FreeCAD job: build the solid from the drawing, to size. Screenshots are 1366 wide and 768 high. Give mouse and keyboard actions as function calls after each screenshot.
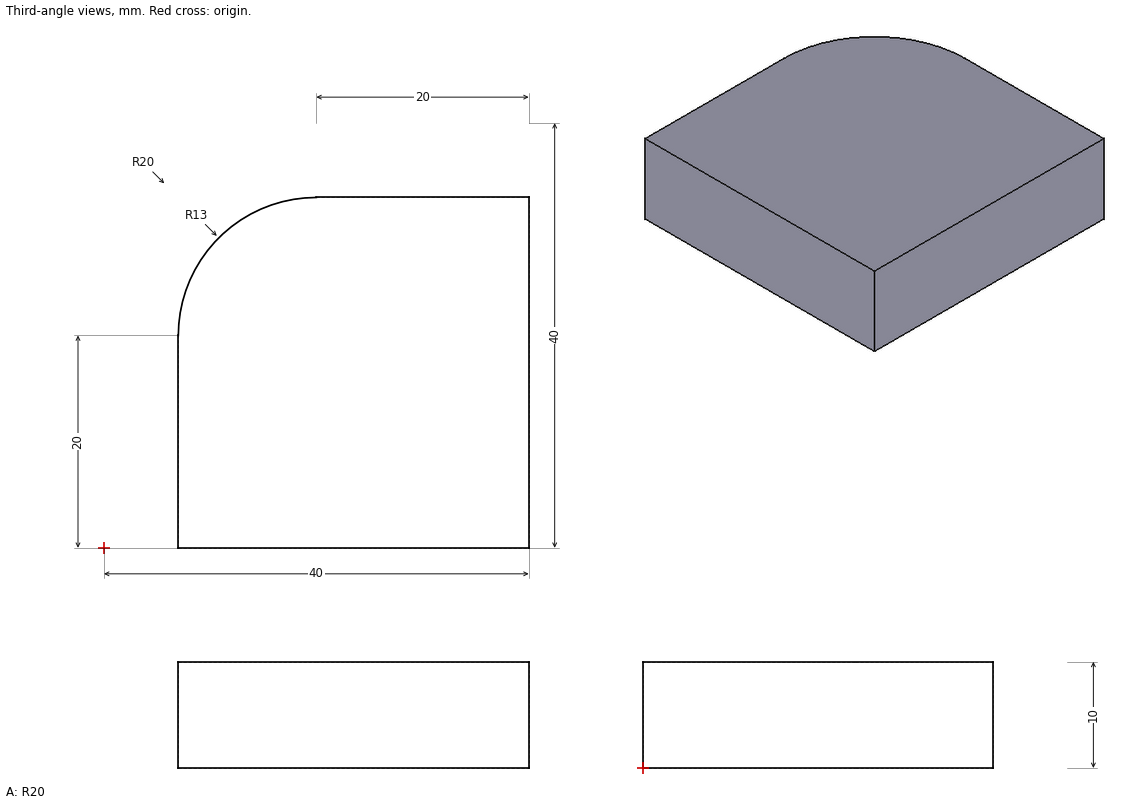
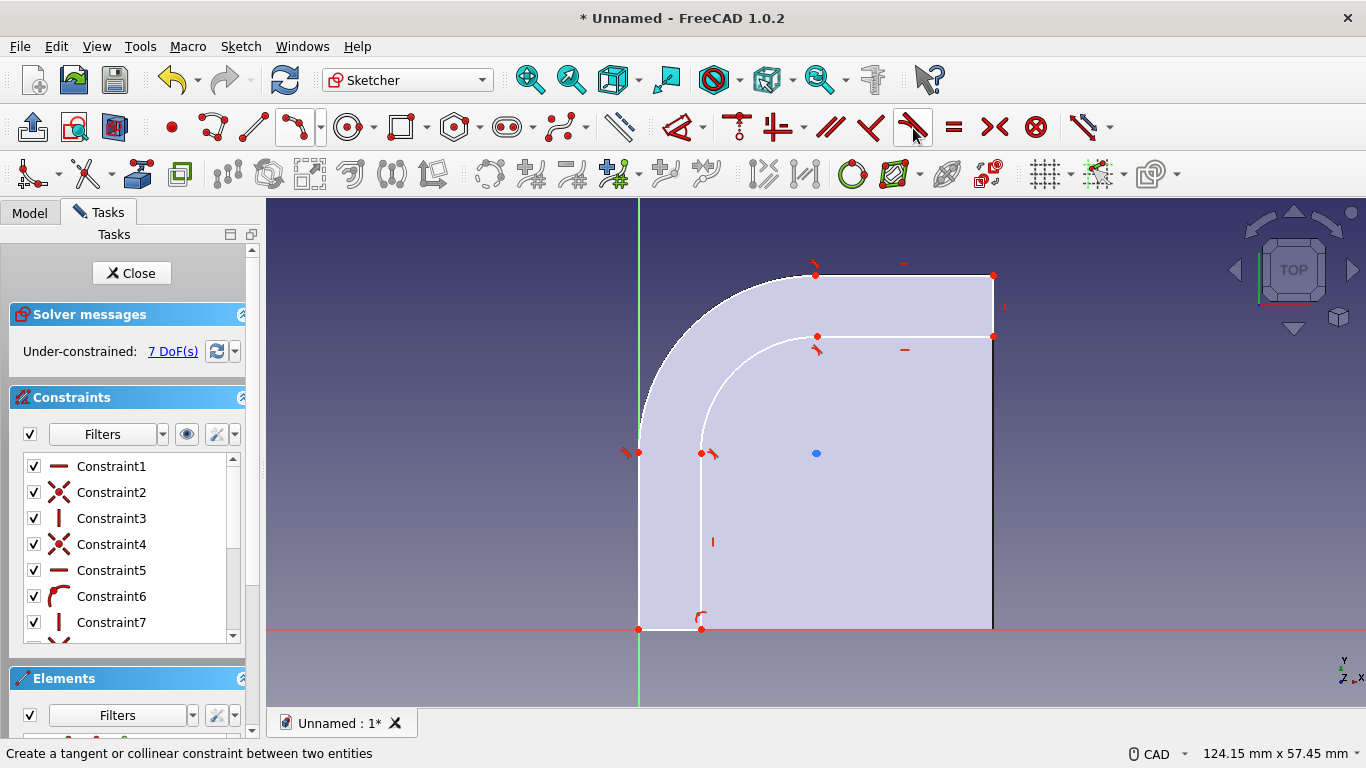
click(639, 577)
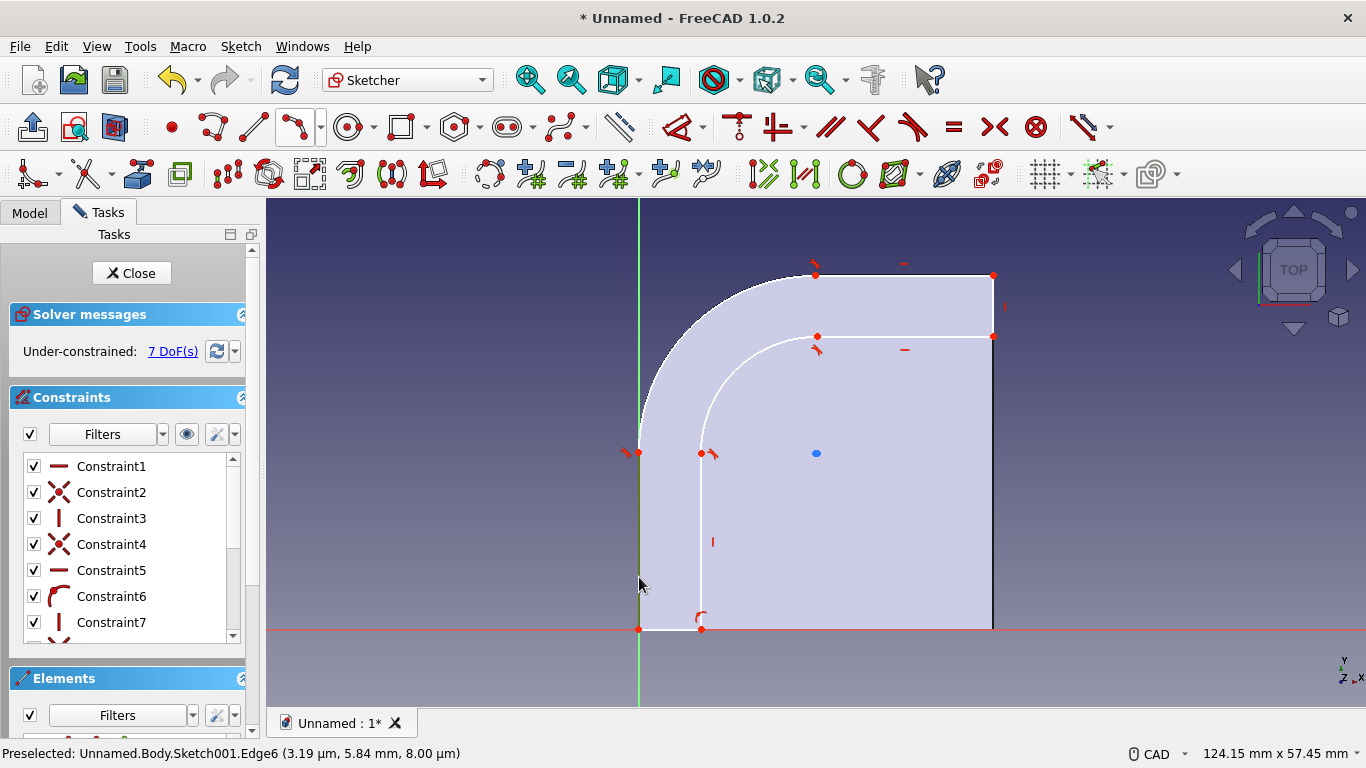
key(v)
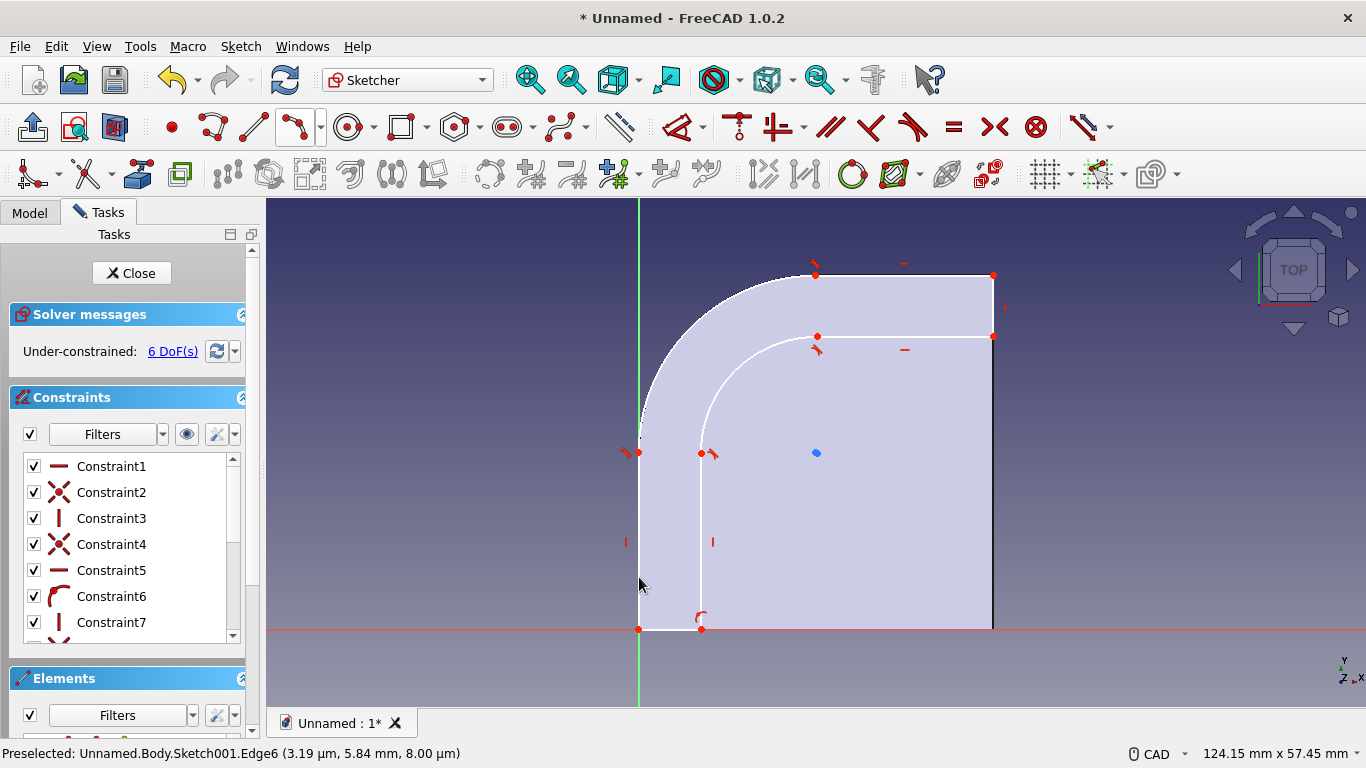
click(764, 350)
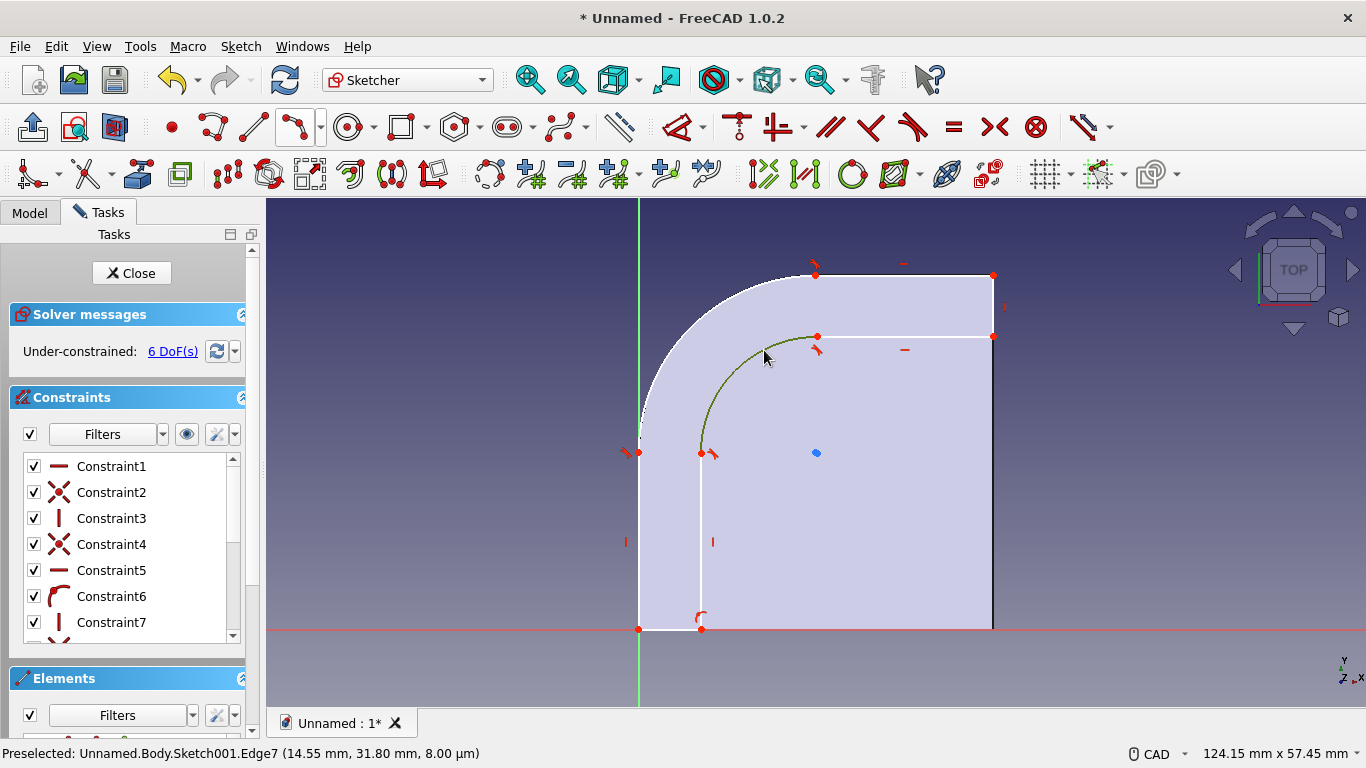
click(736, 295)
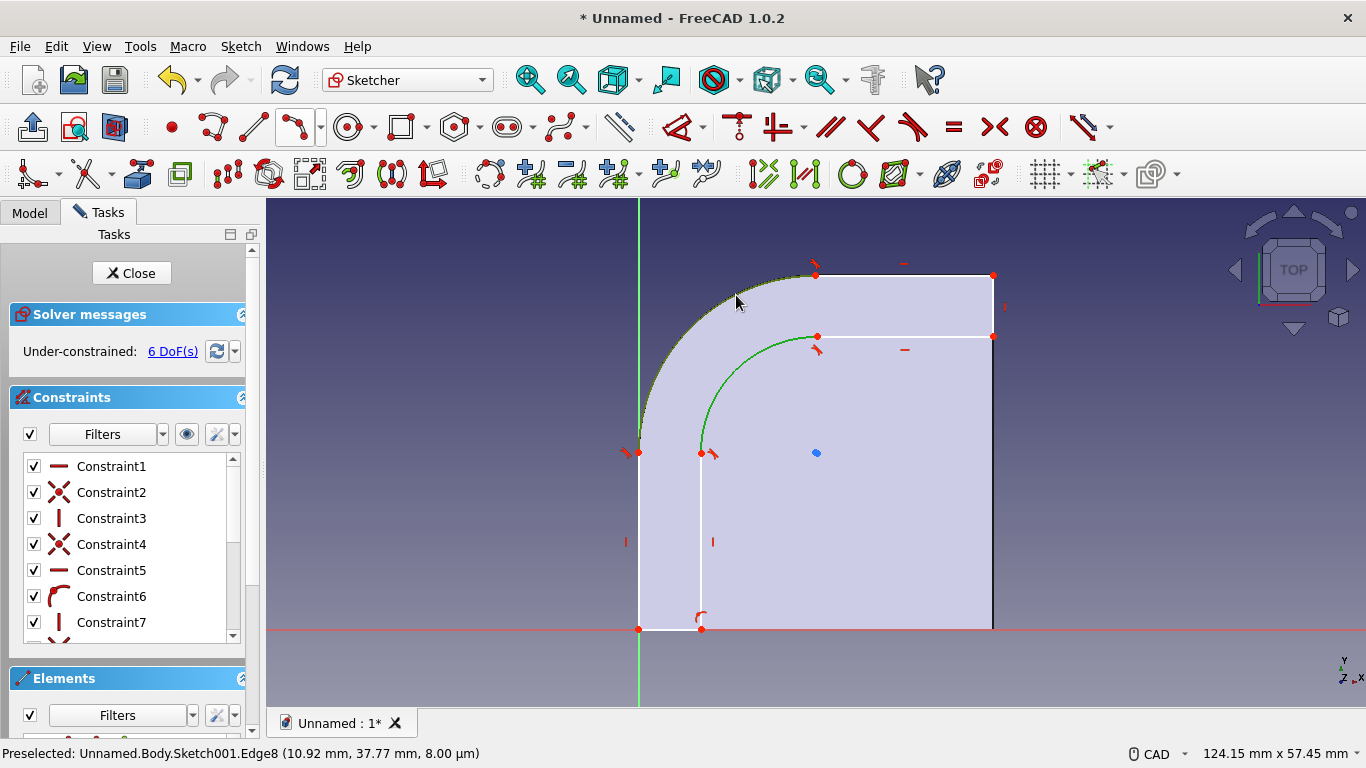
click(737, 128)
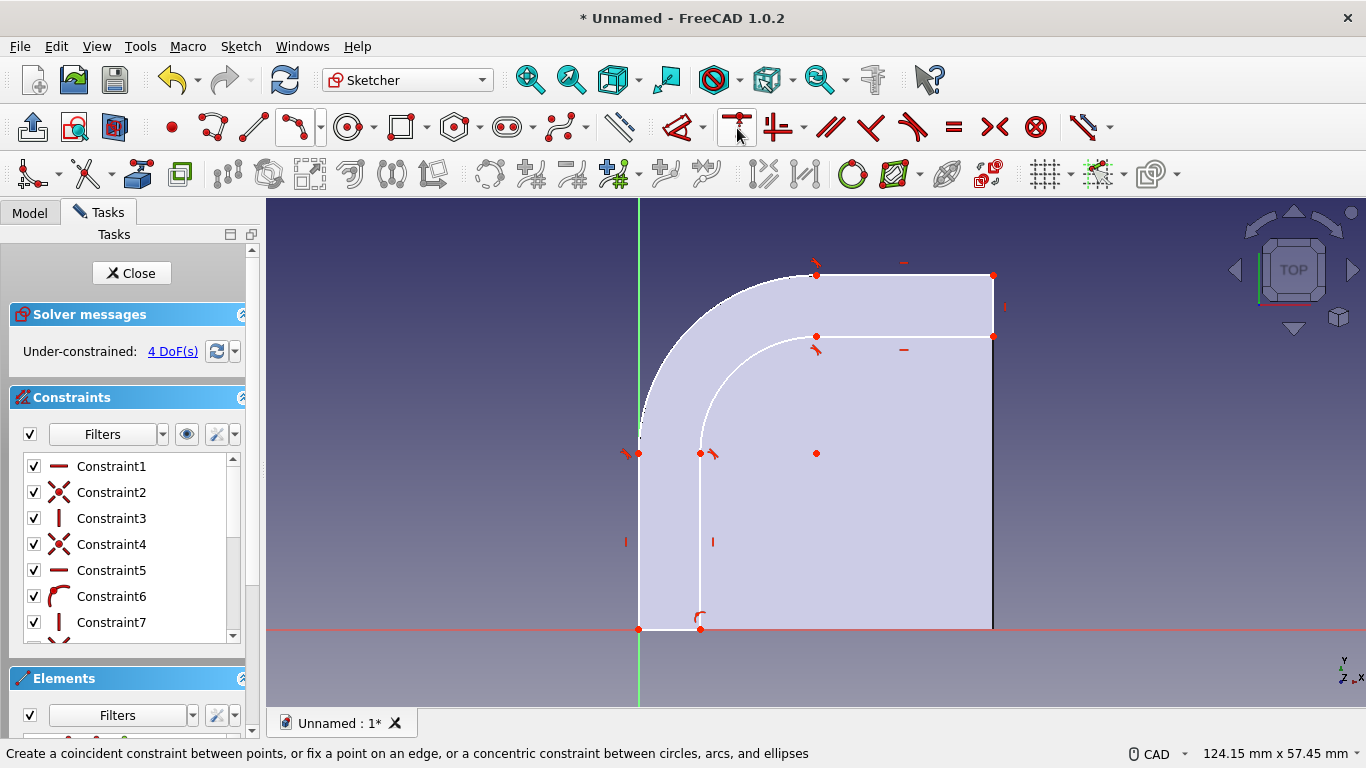
click(676, 128)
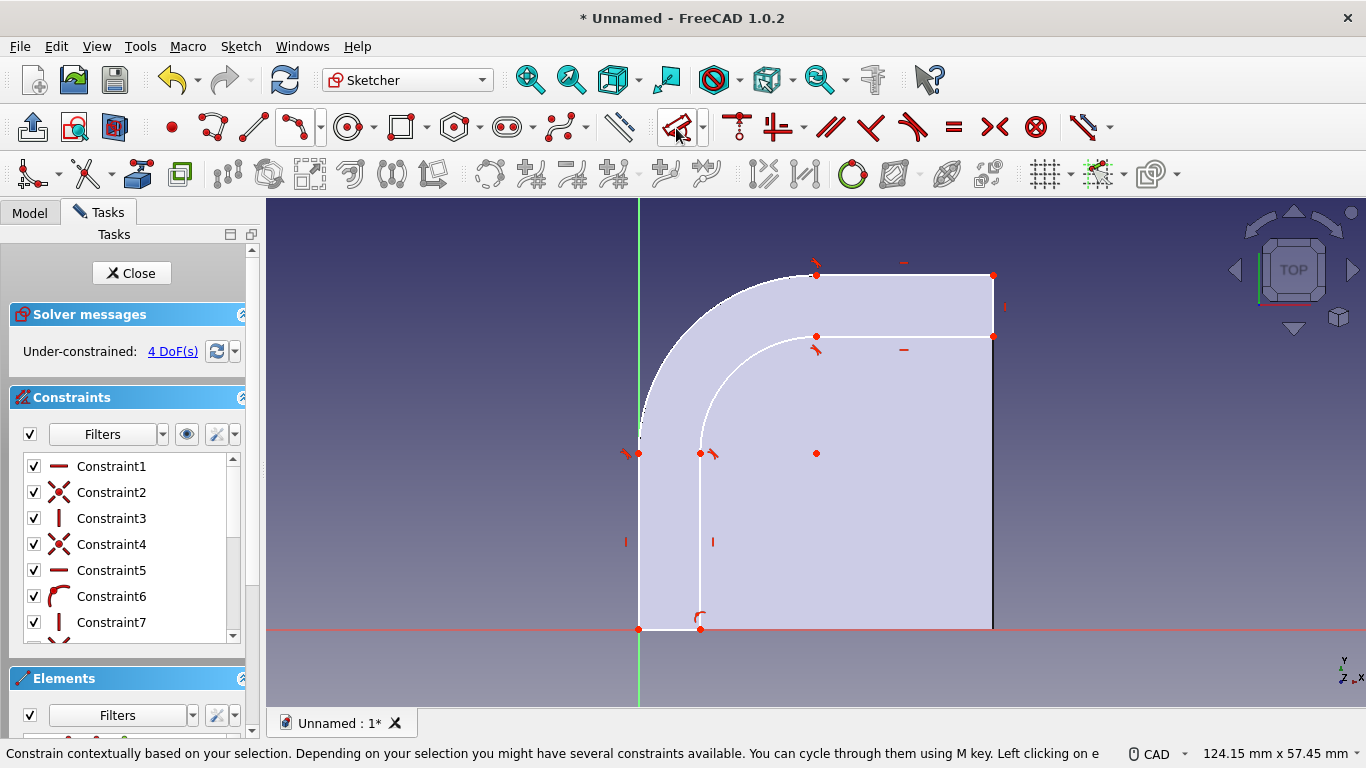
click(764, 350)
click(749, 321)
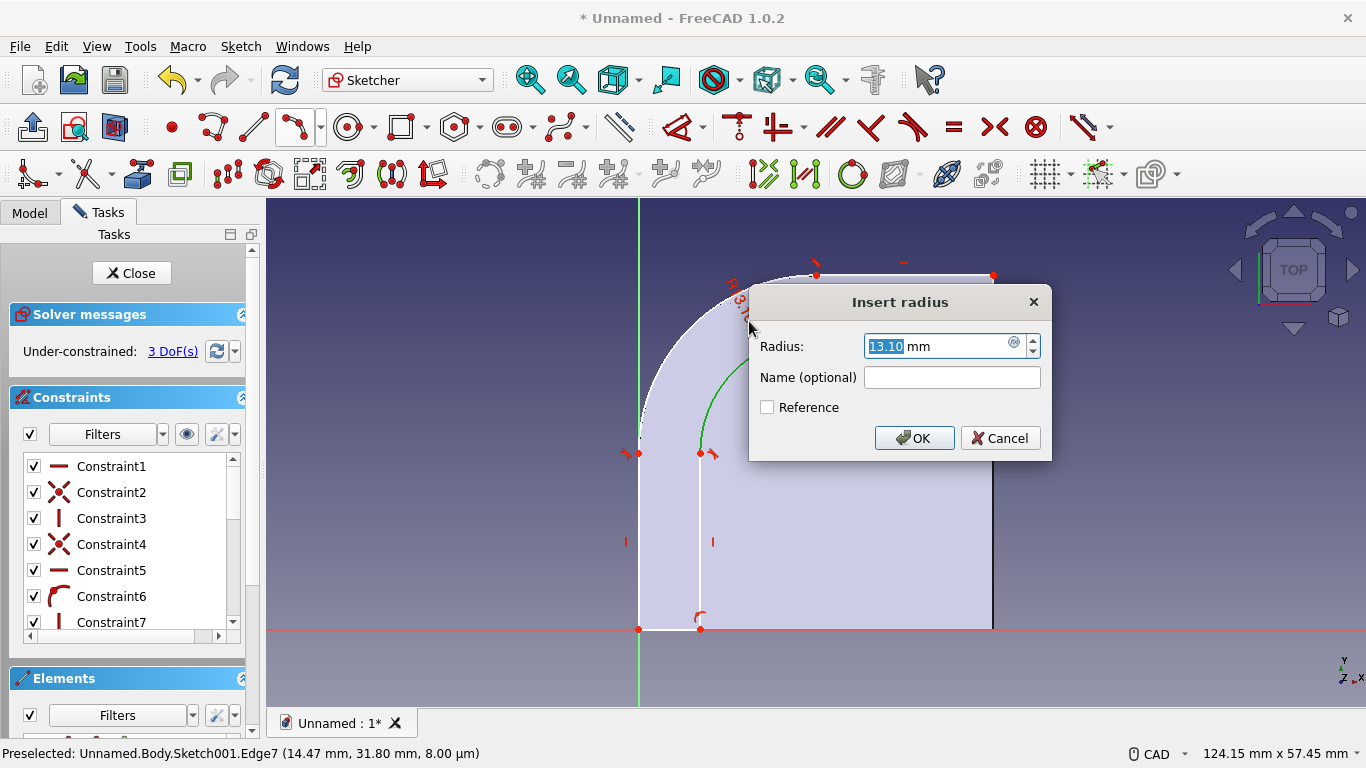
text(13)
key(Return)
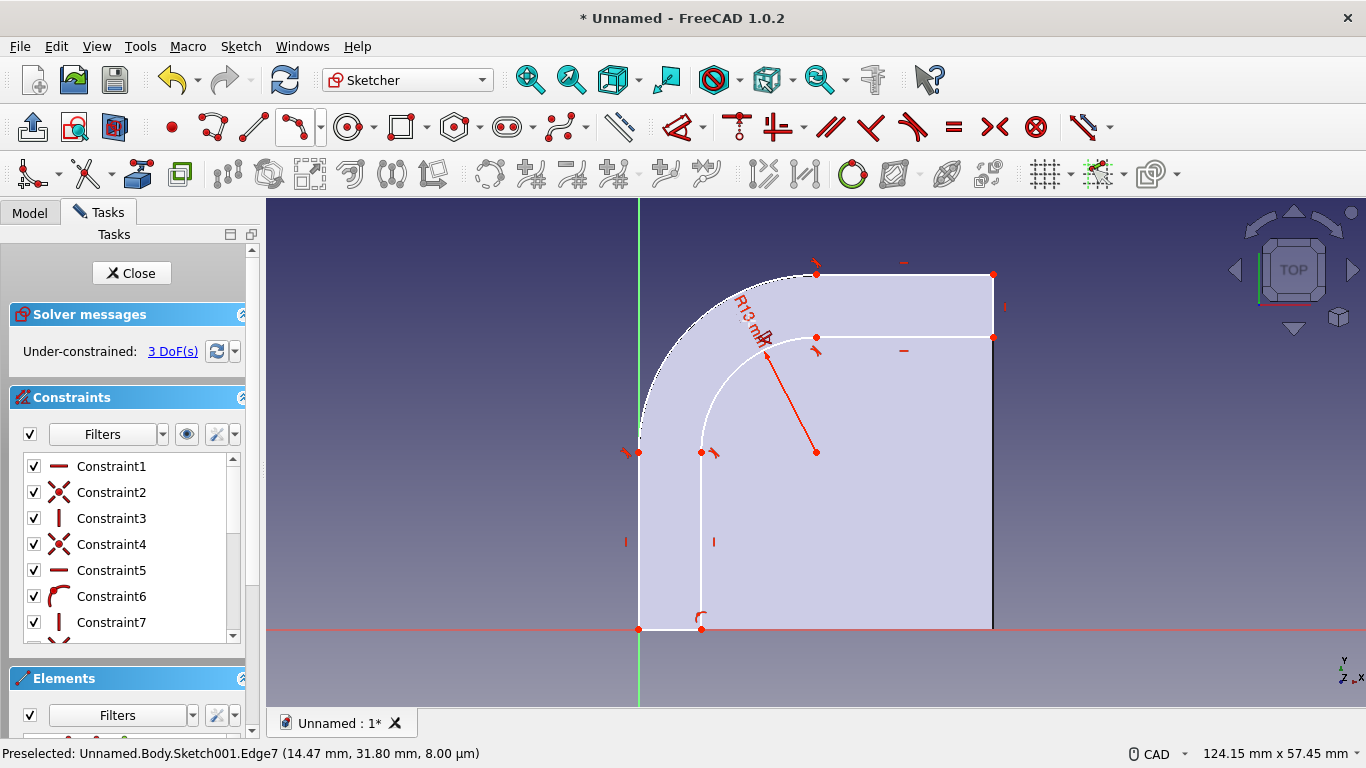
click(736, 294)
click(722, 265)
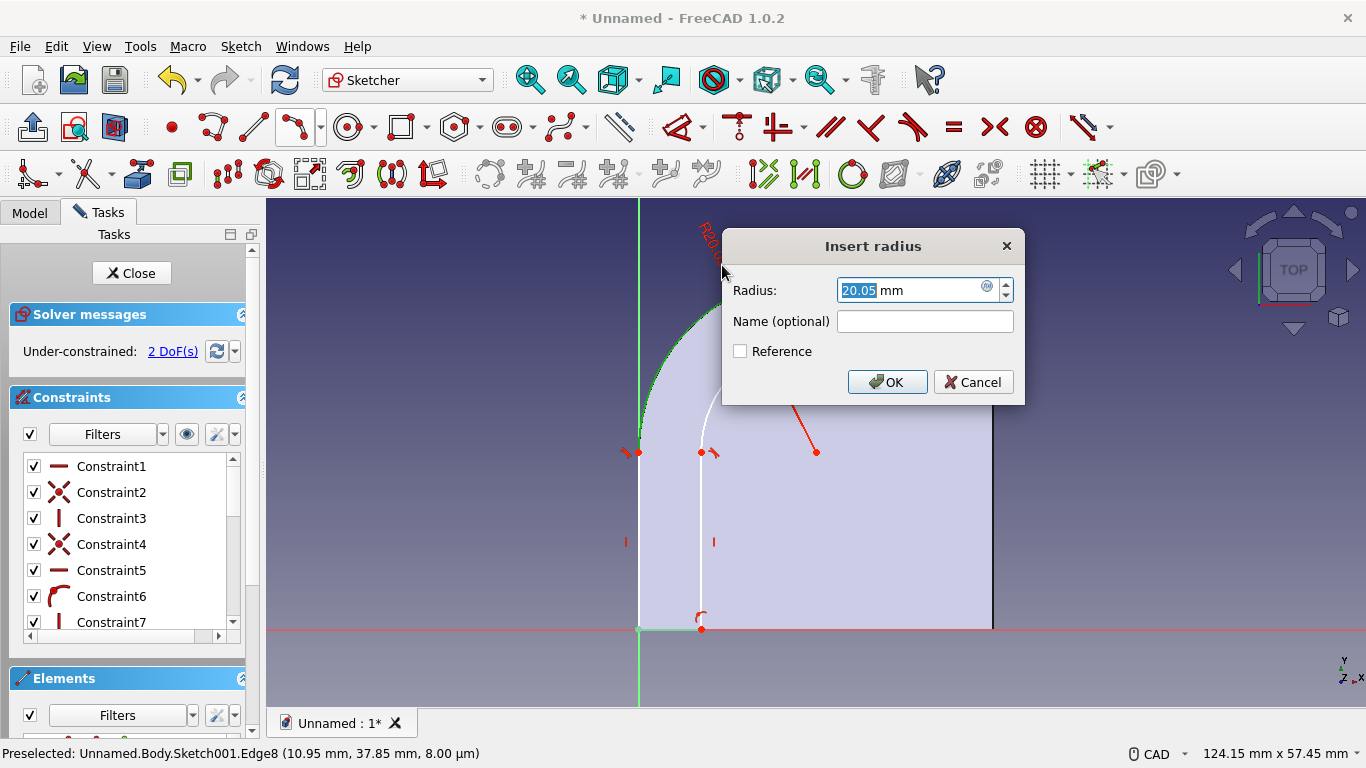
text(20)
key(Return)